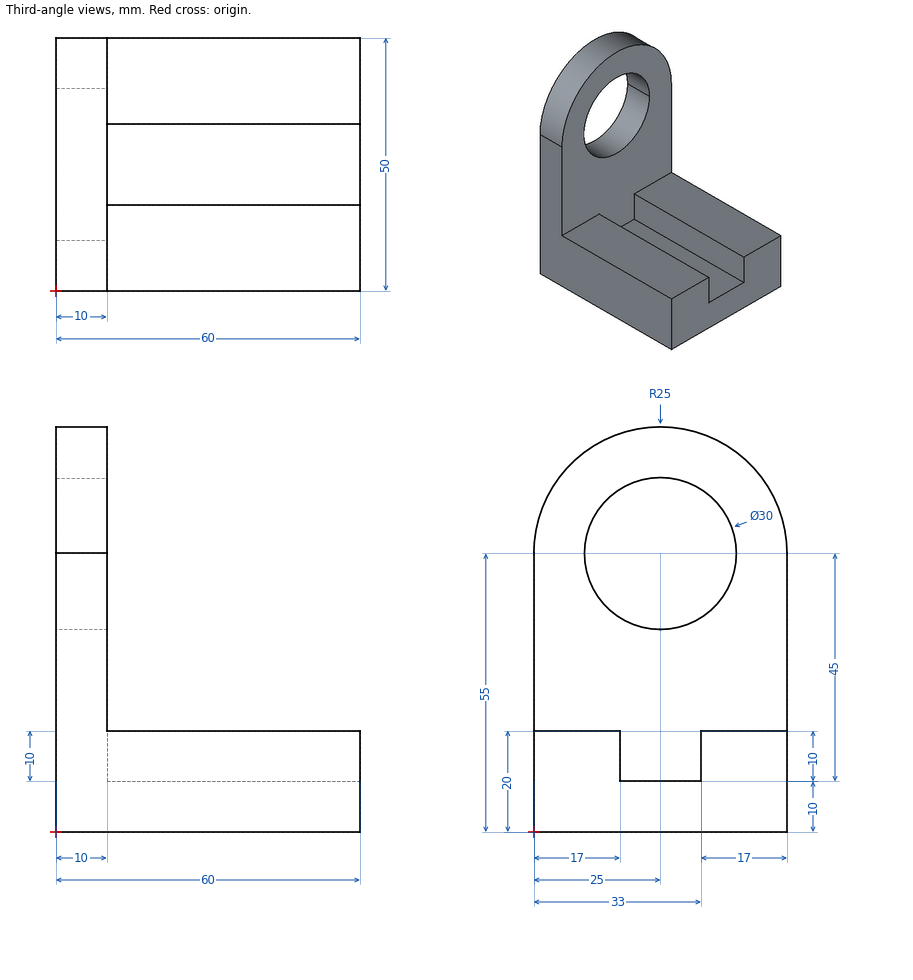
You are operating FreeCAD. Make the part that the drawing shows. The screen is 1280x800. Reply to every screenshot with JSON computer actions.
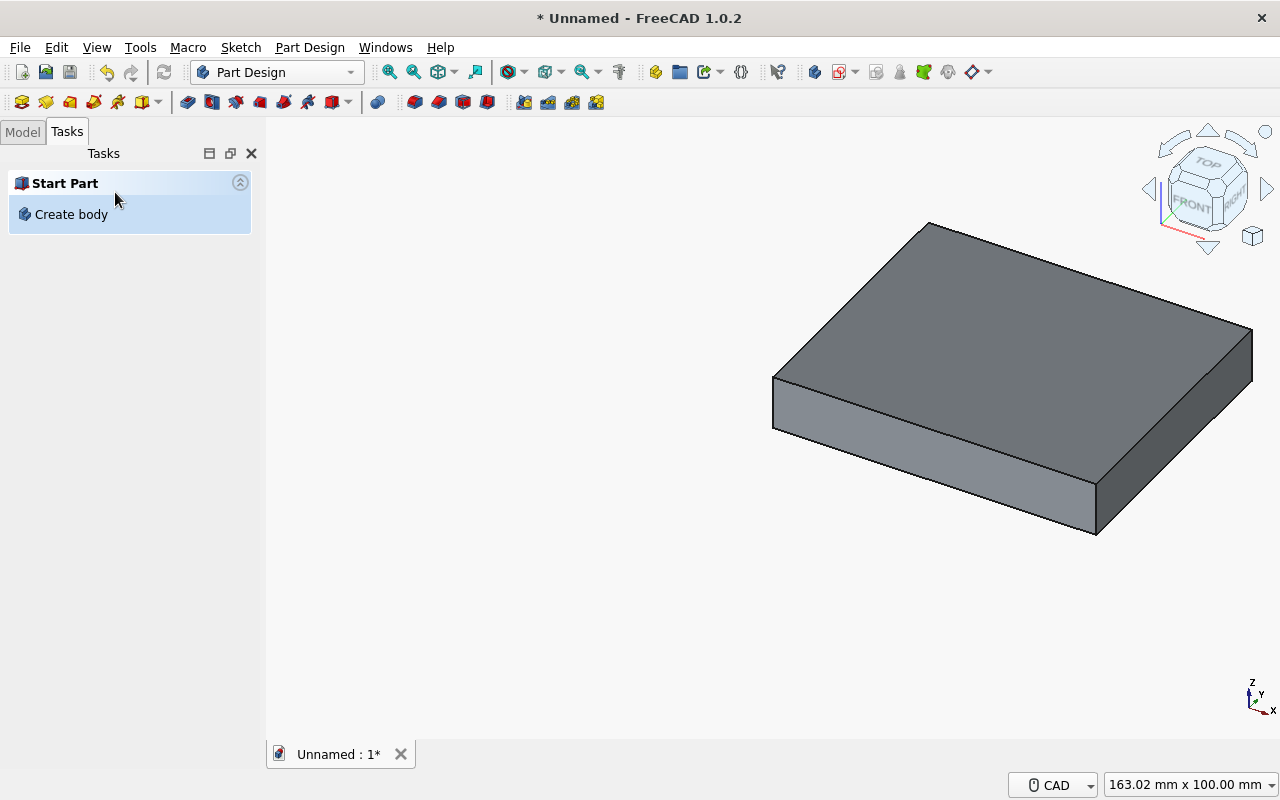
{"action": "left_click", "coordinate": [1196, 409]}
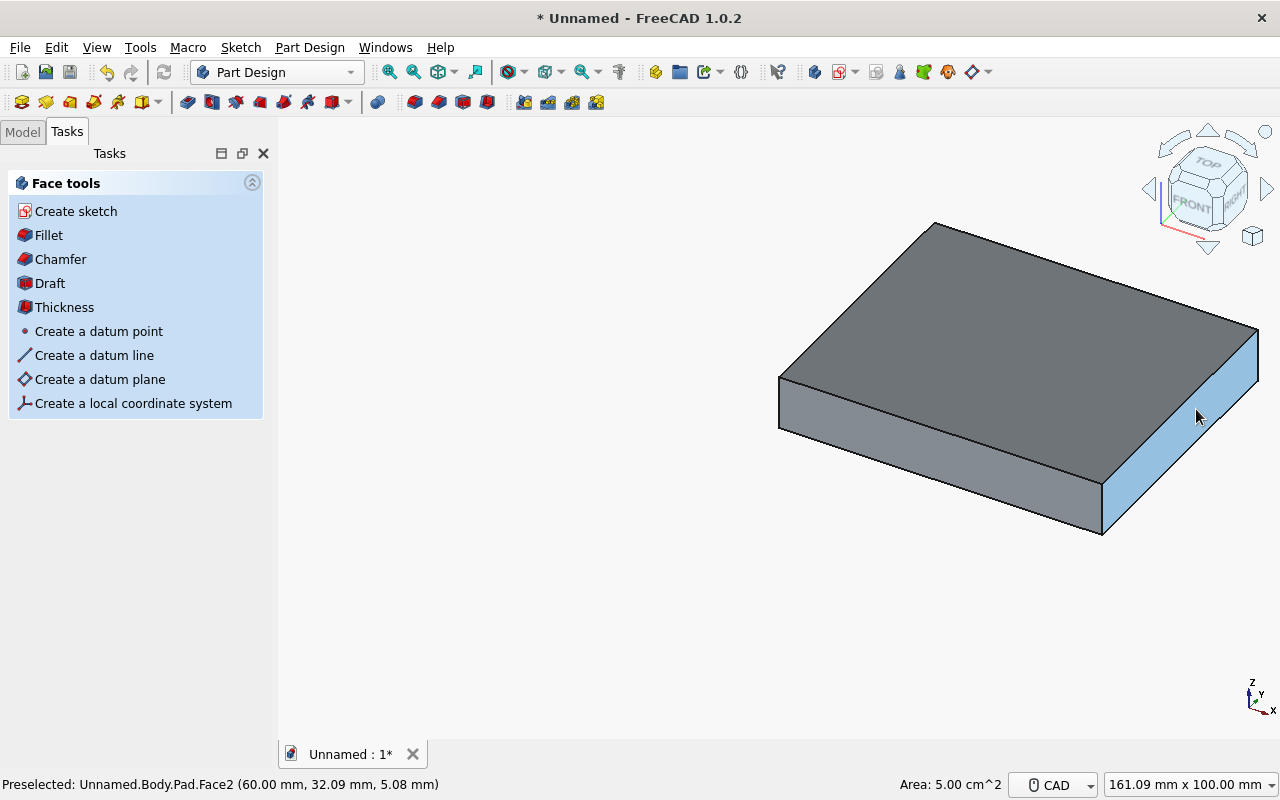
{"action": "left_click", "coordinate": [840, 72]}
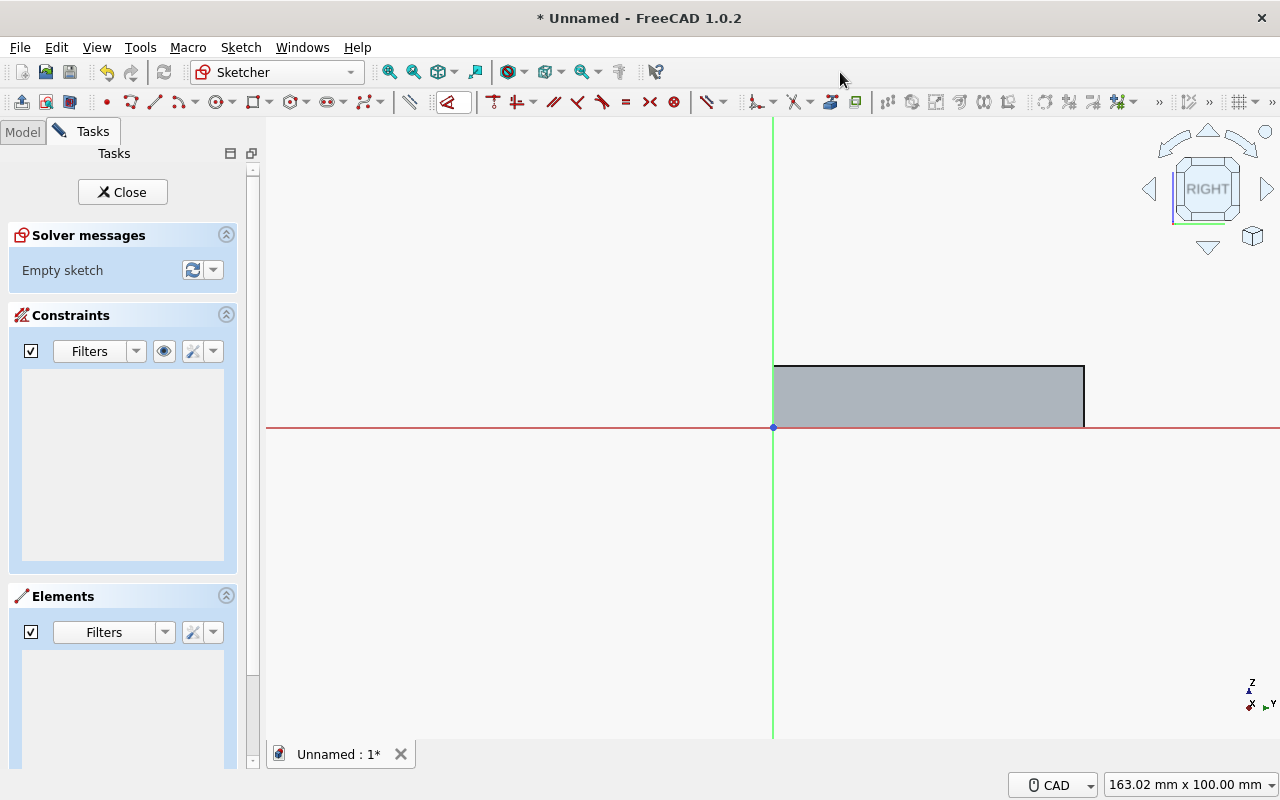
{"action": "scroll", "coordinate": [1115, 290], "scroll_direction": "up", "scroll_amount": 3}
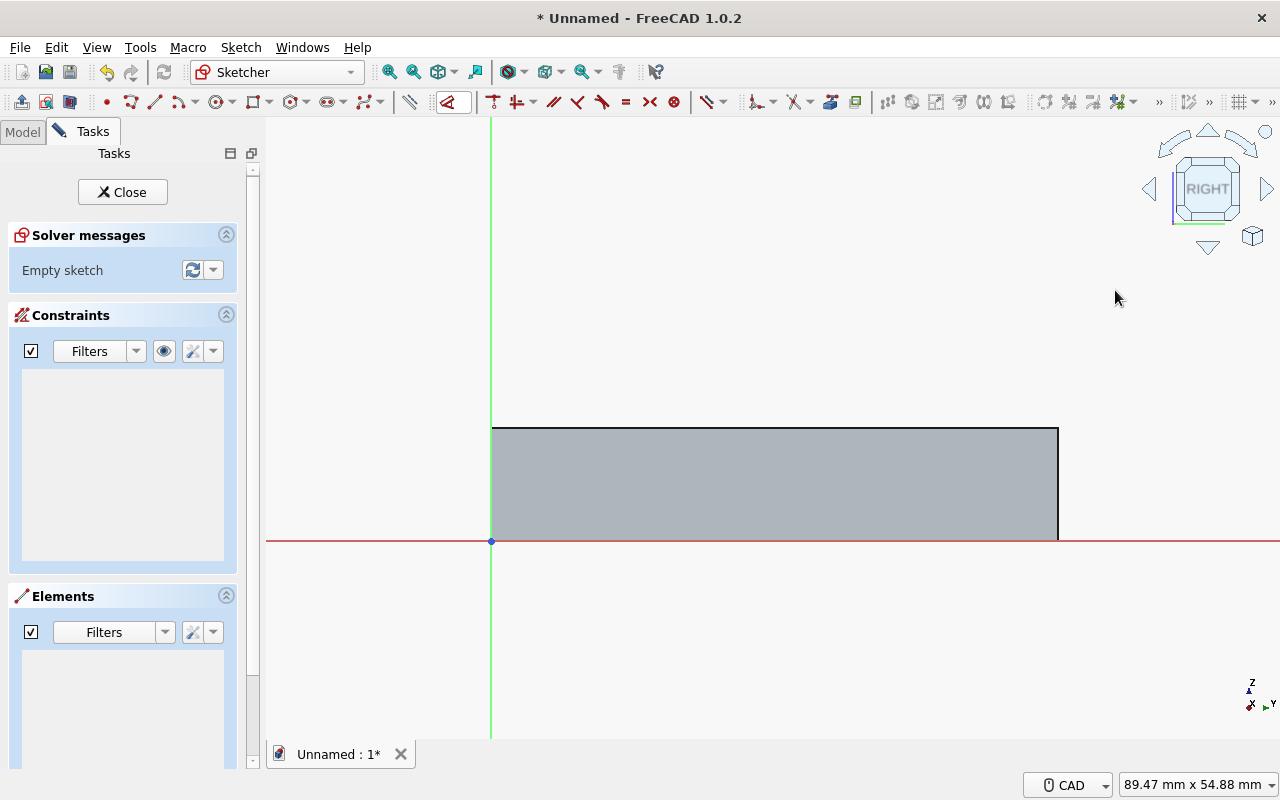
{"action": "left_click", "coordinate": [254, 102]}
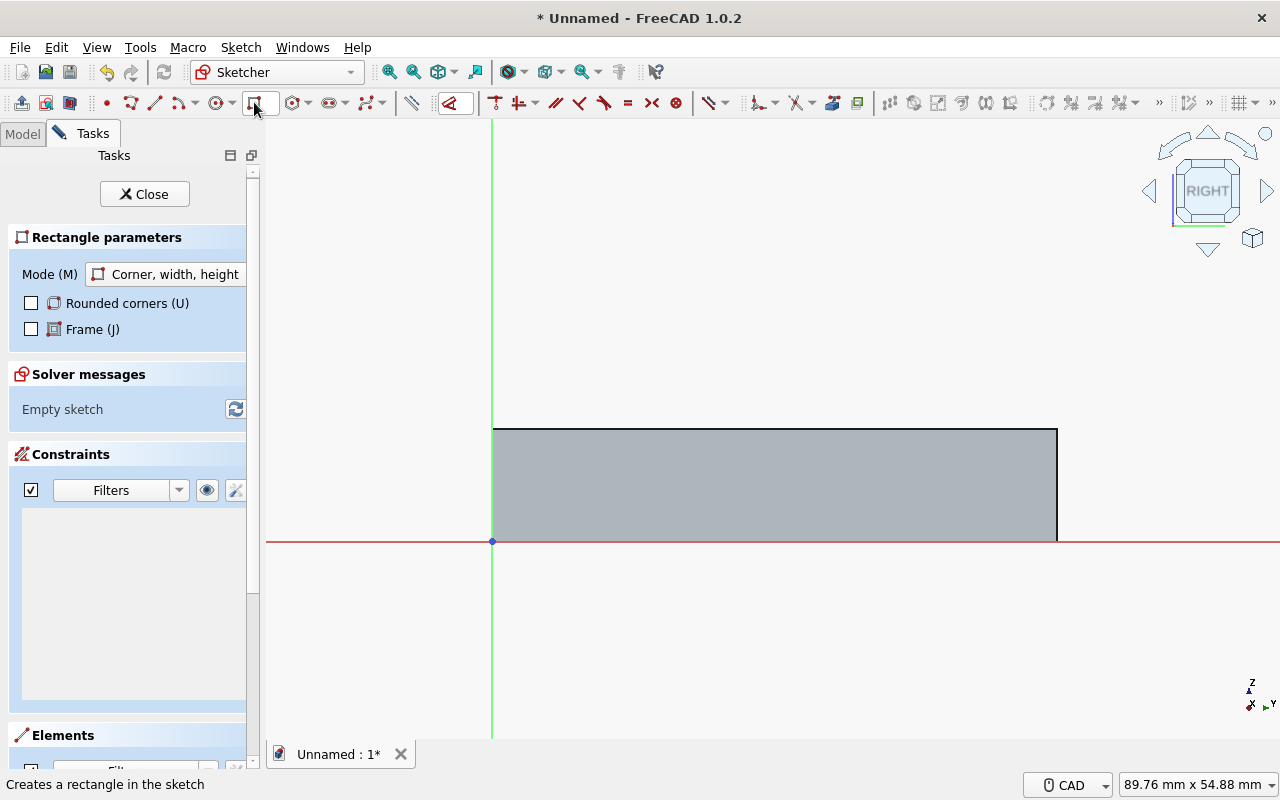
{"action": "left_click", "coordinate": [865, 316]}
{"action": "left_click", "coordinate": [1057, 429]}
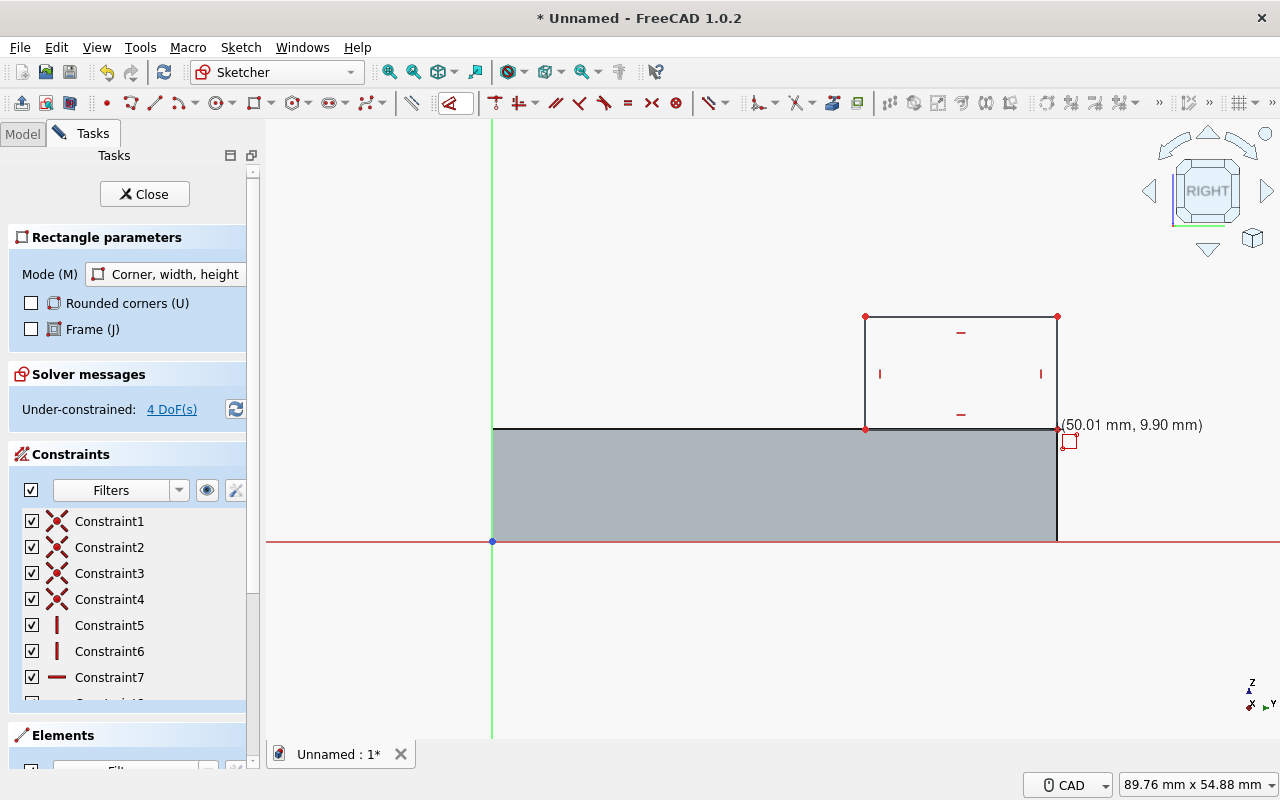
{"action": "left_click", "coordinate": [492, 316]}
{"action": "left_click", "coordinate": [684, 429]}
{"action": "key", "text": "Escape"}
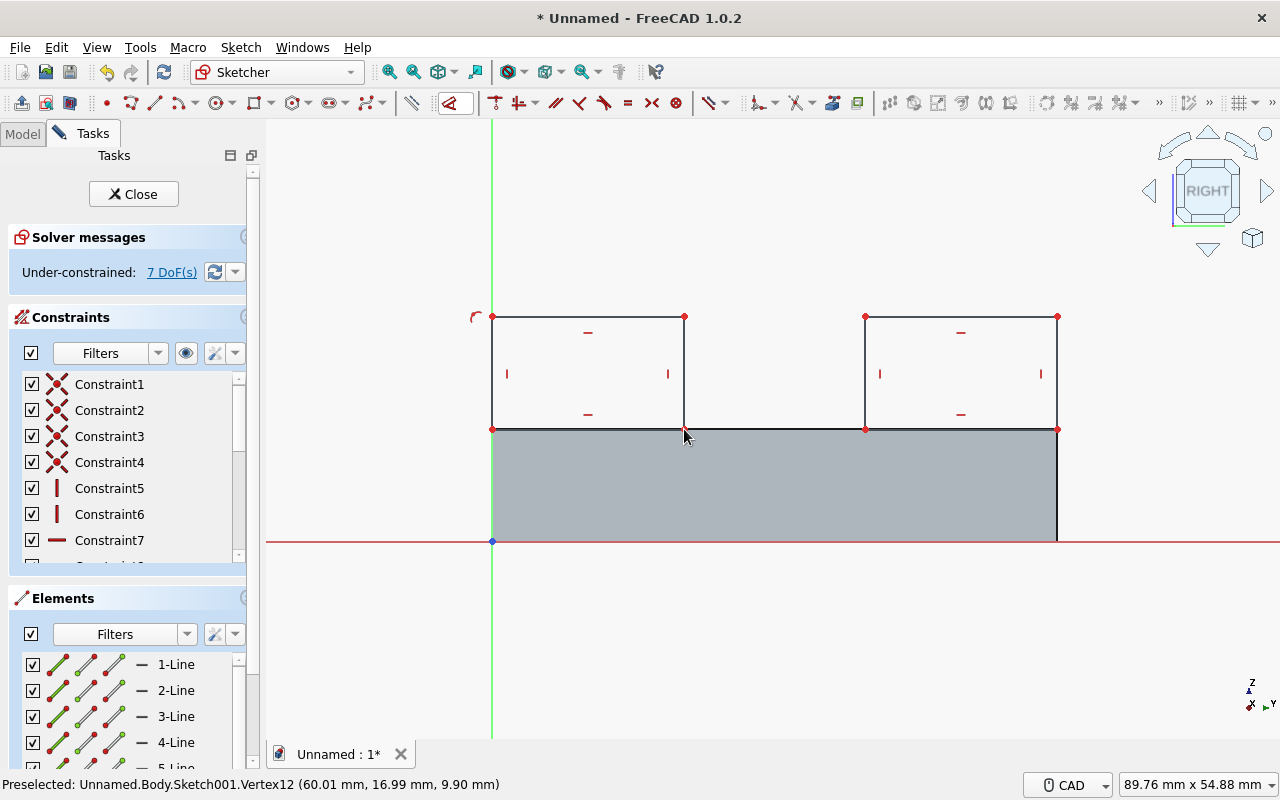
{"action": "left_click", "coordinate": [865, 351]}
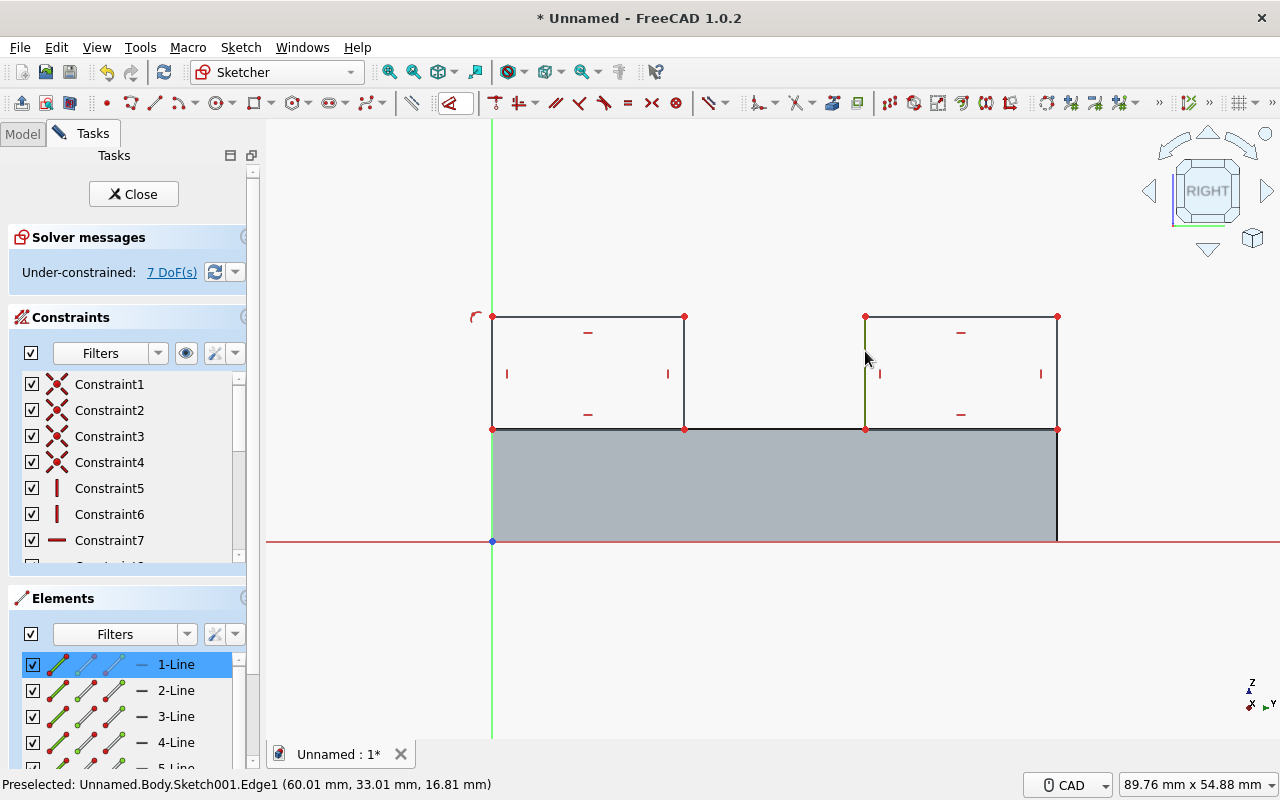
{"action": "key", "text": "i"}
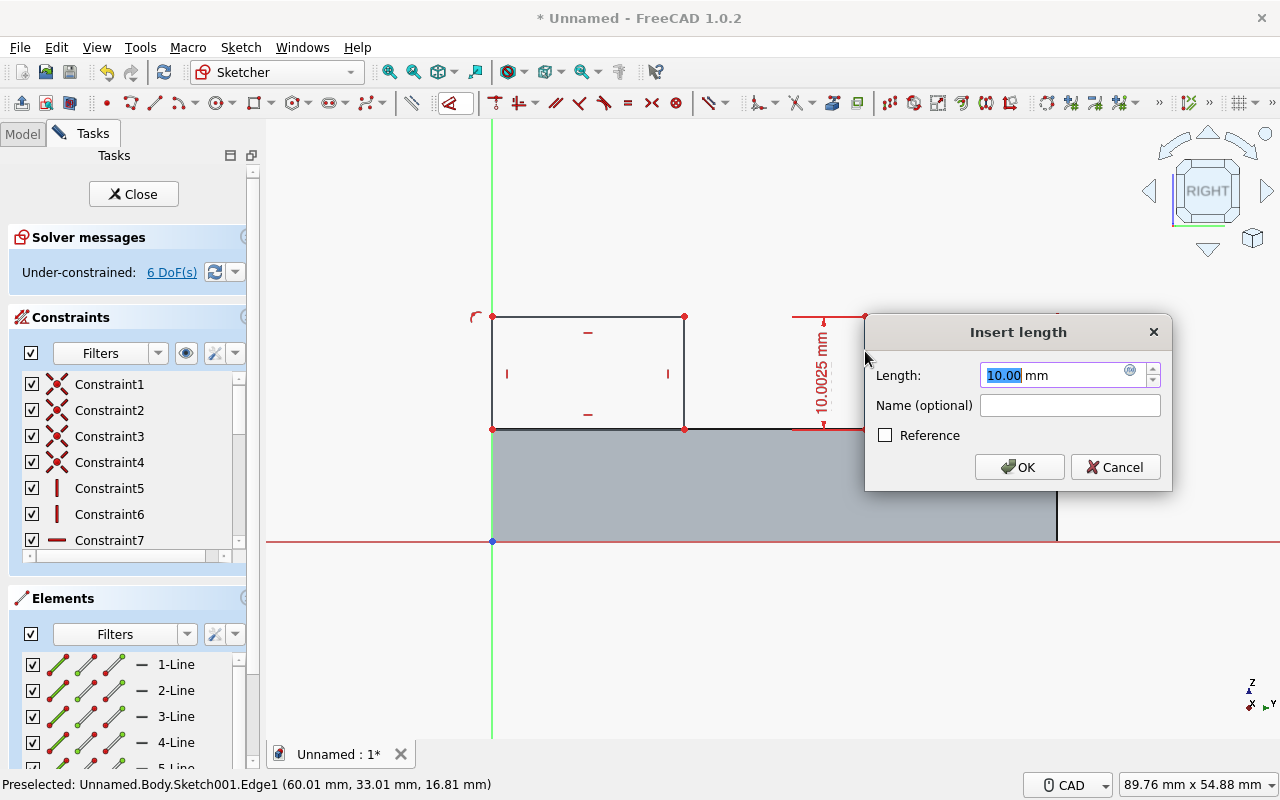
{"action": "type", "text": "10"}
{"action": "key", "text": "Return"}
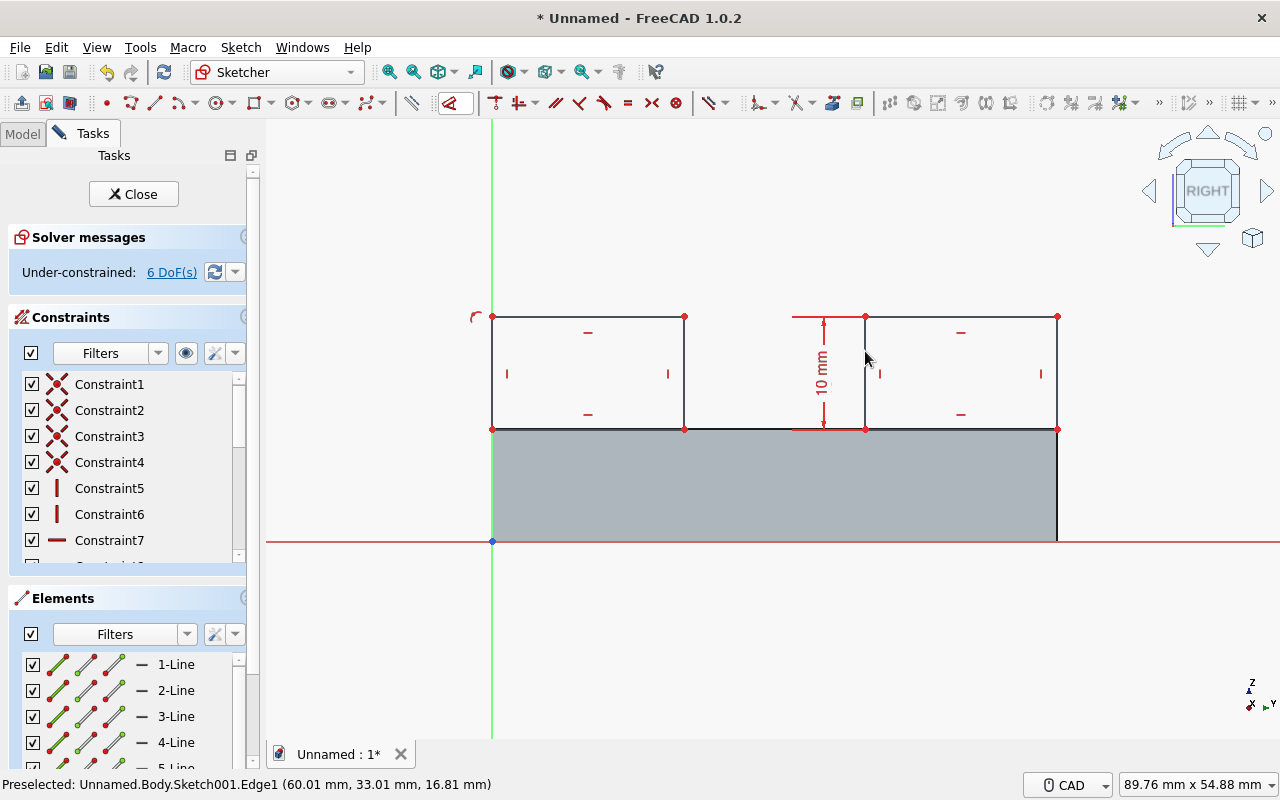
{"action": "left_click", "coordinate": [923, 430]}